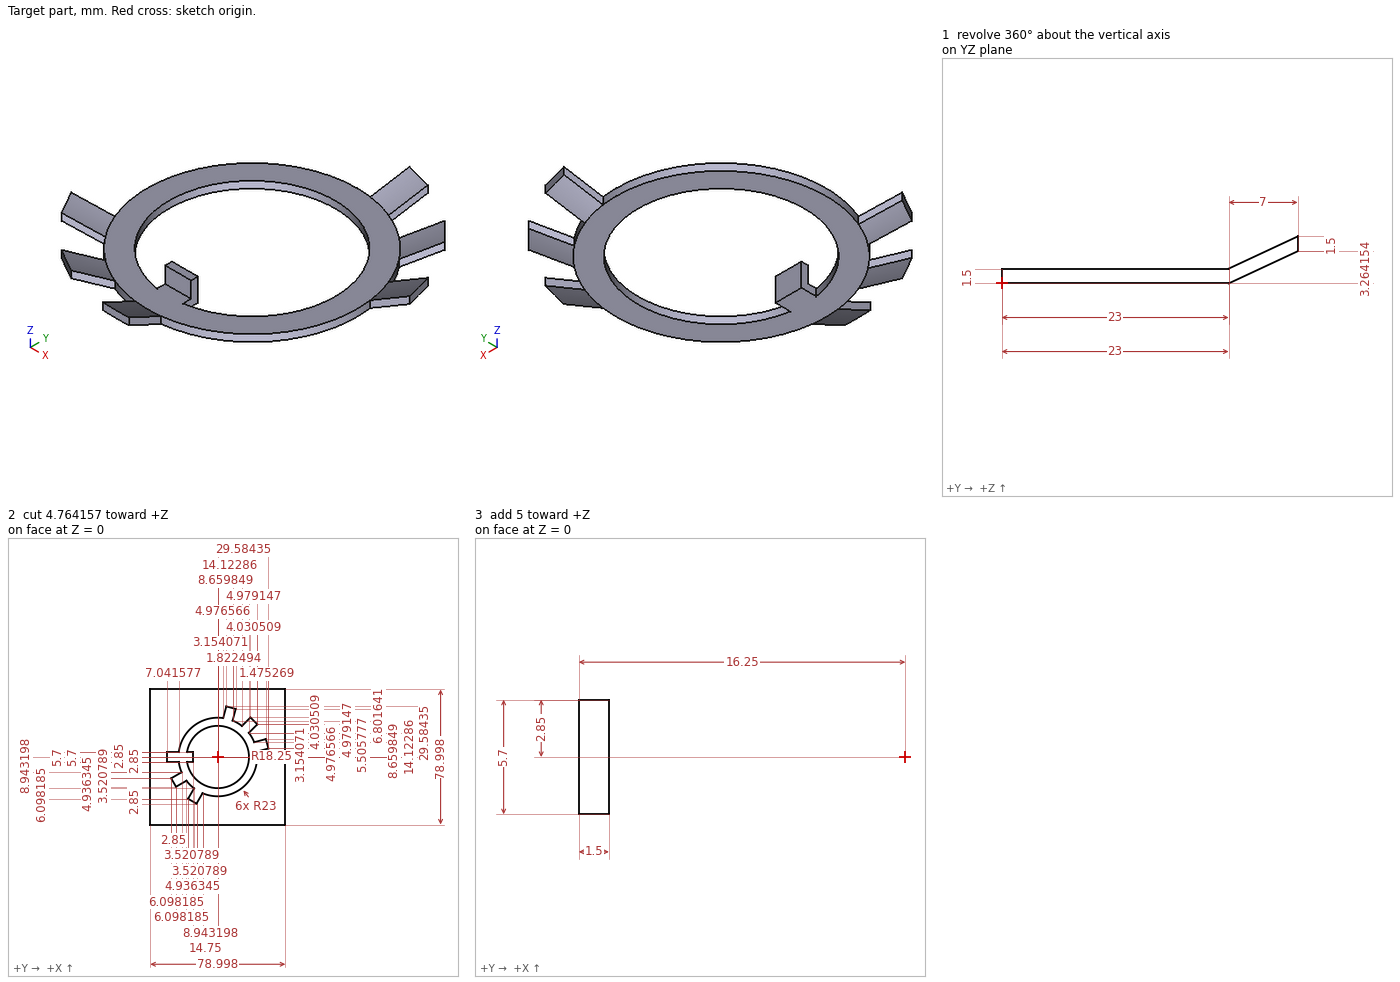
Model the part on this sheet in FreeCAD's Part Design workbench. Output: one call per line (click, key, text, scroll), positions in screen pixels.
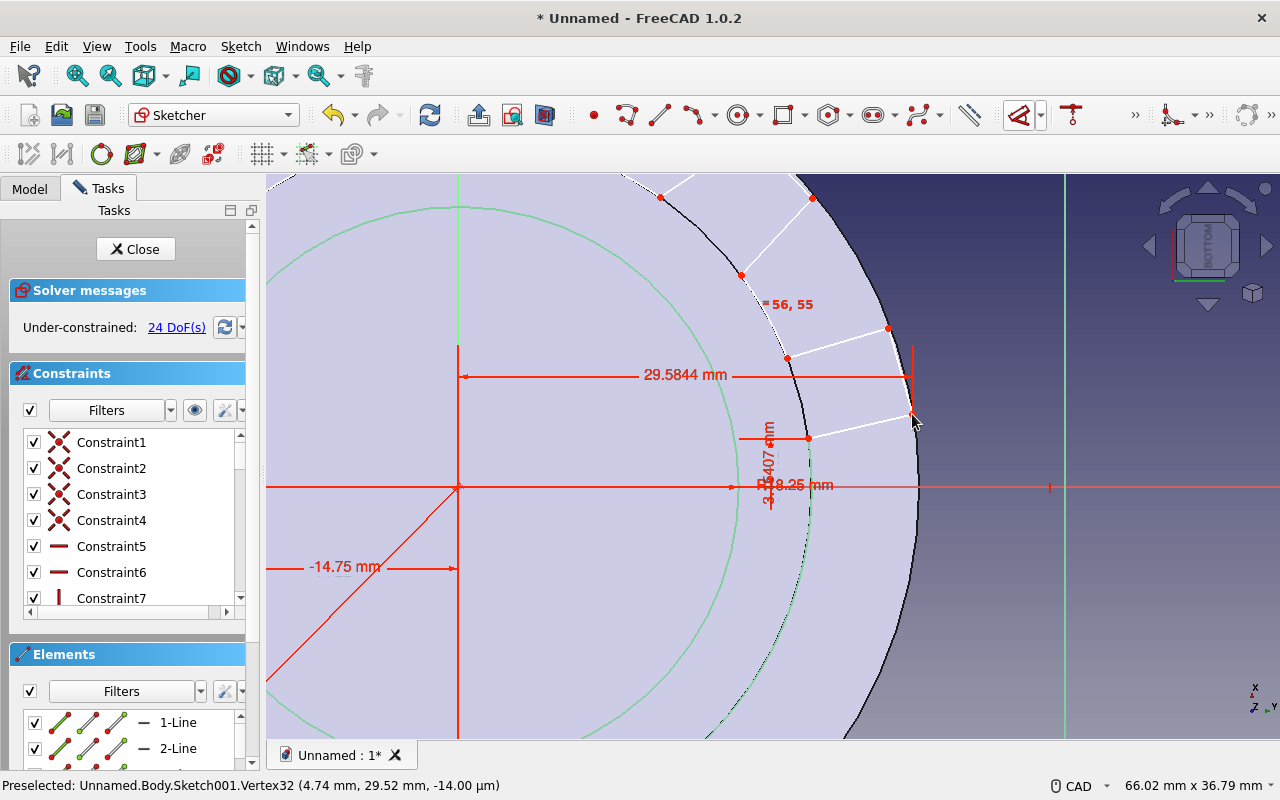
click(913, 414)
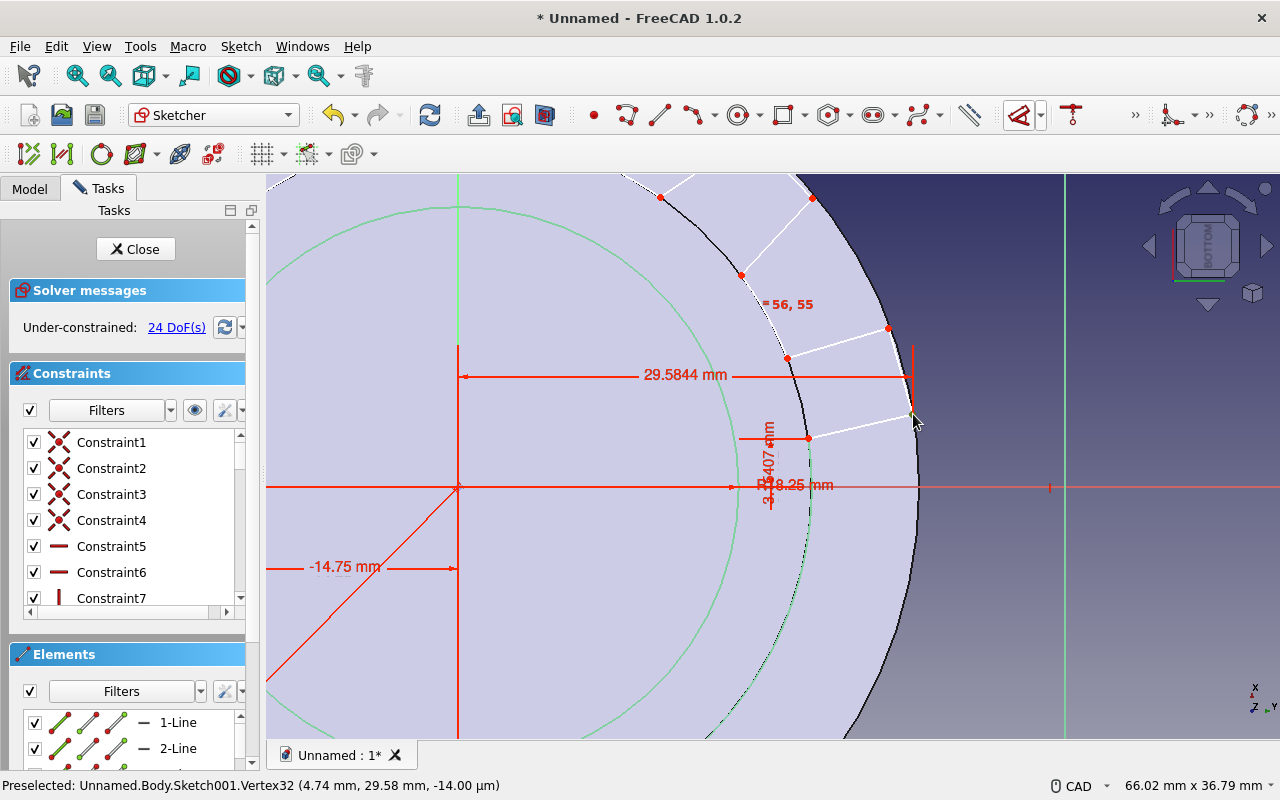
click(1040, 116)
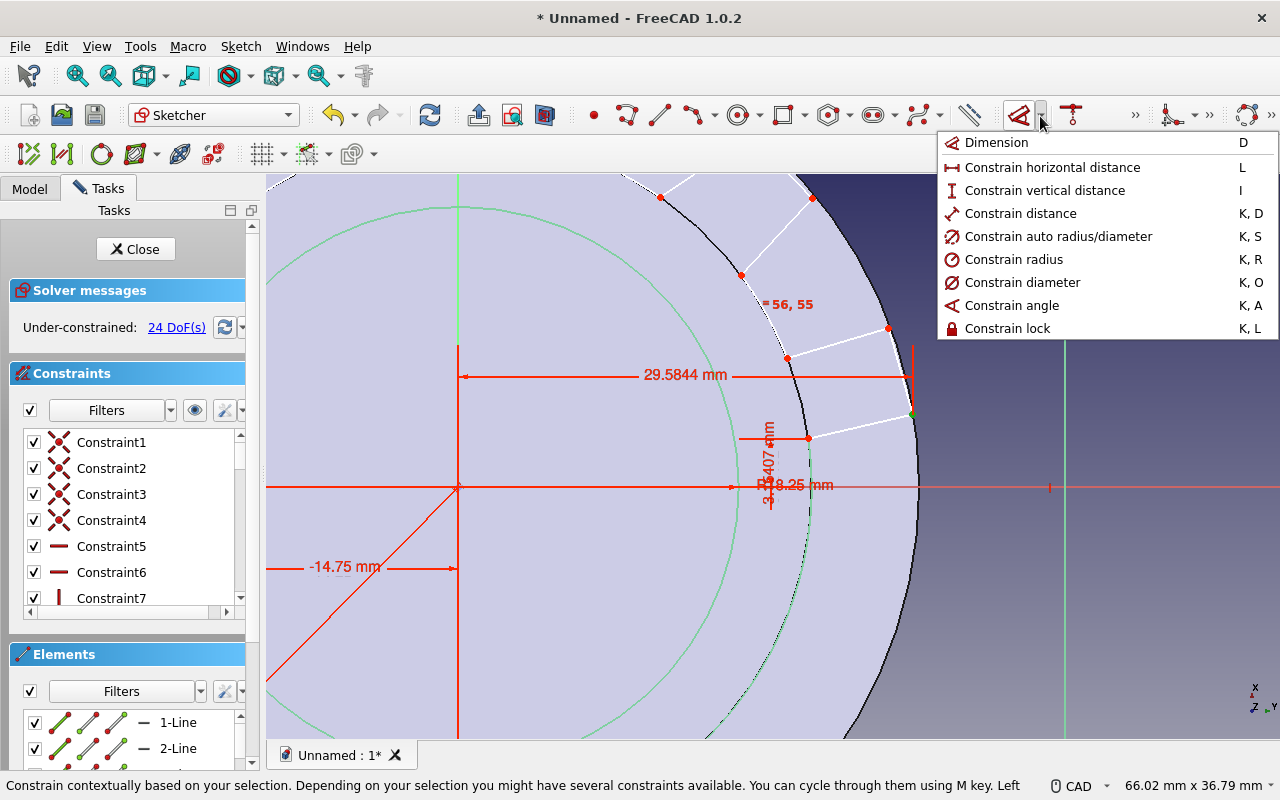
click(1108, 190)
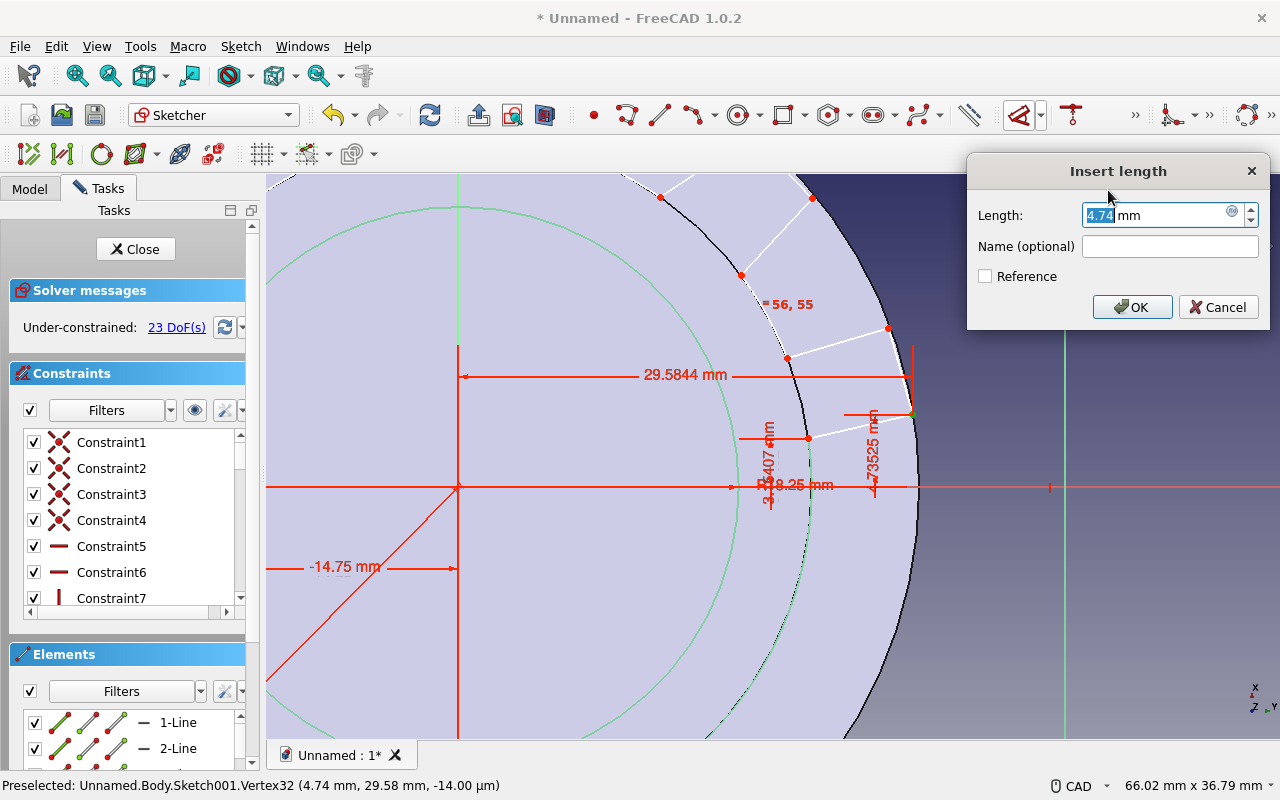
text(4.976566)
key(Return)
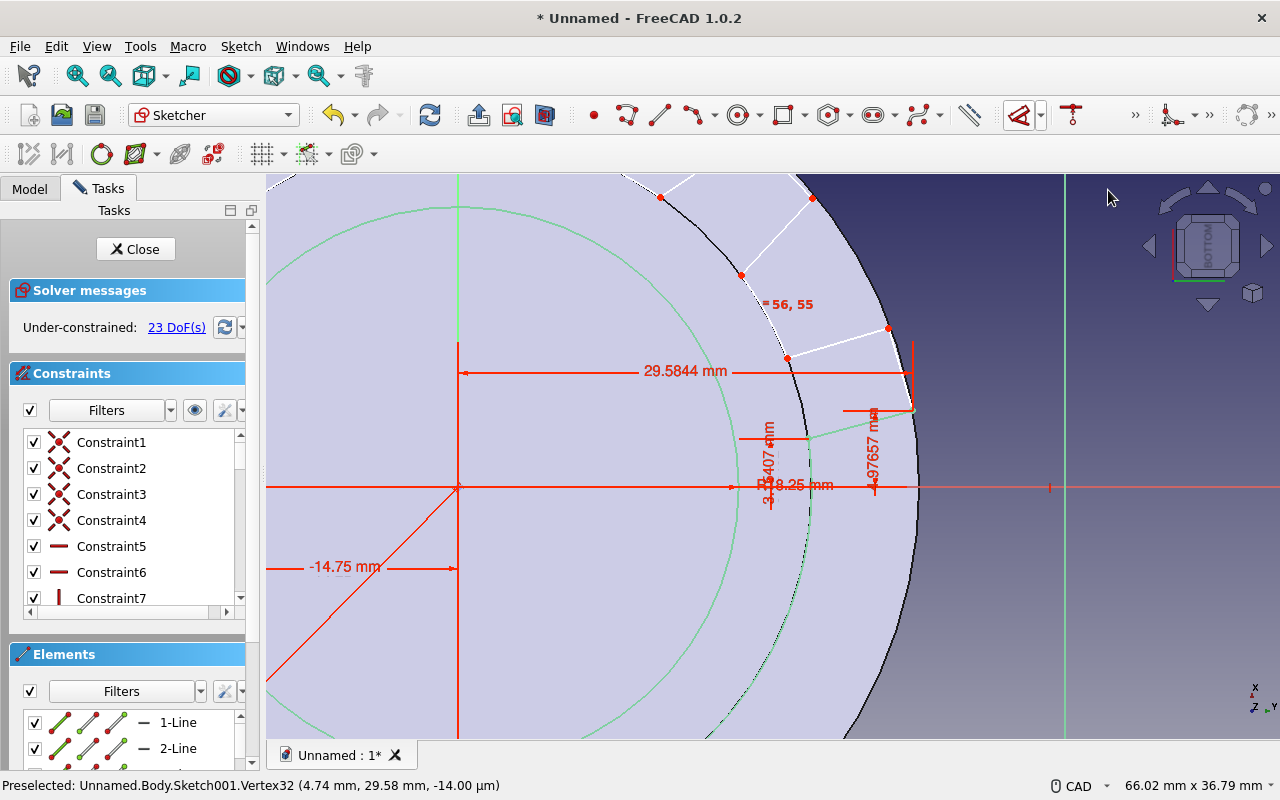
click(787, 358)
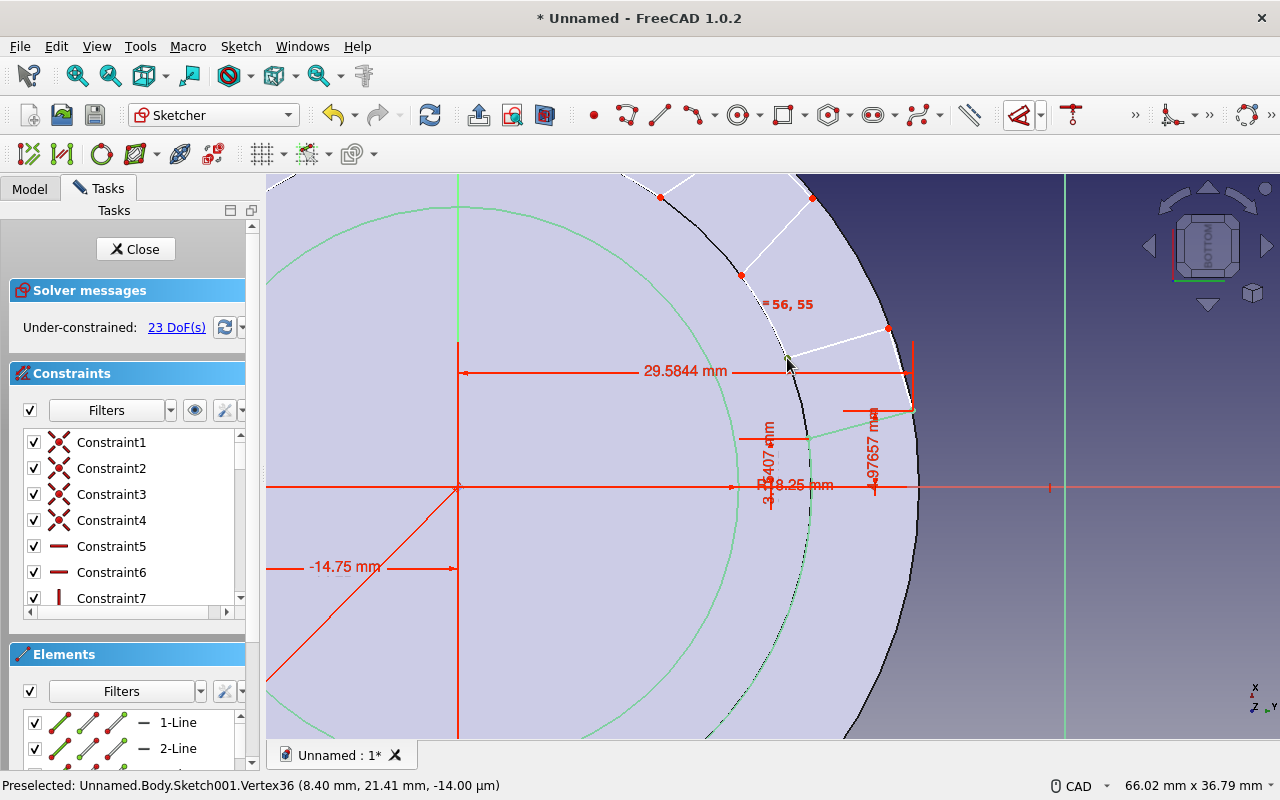
click(1040, 116)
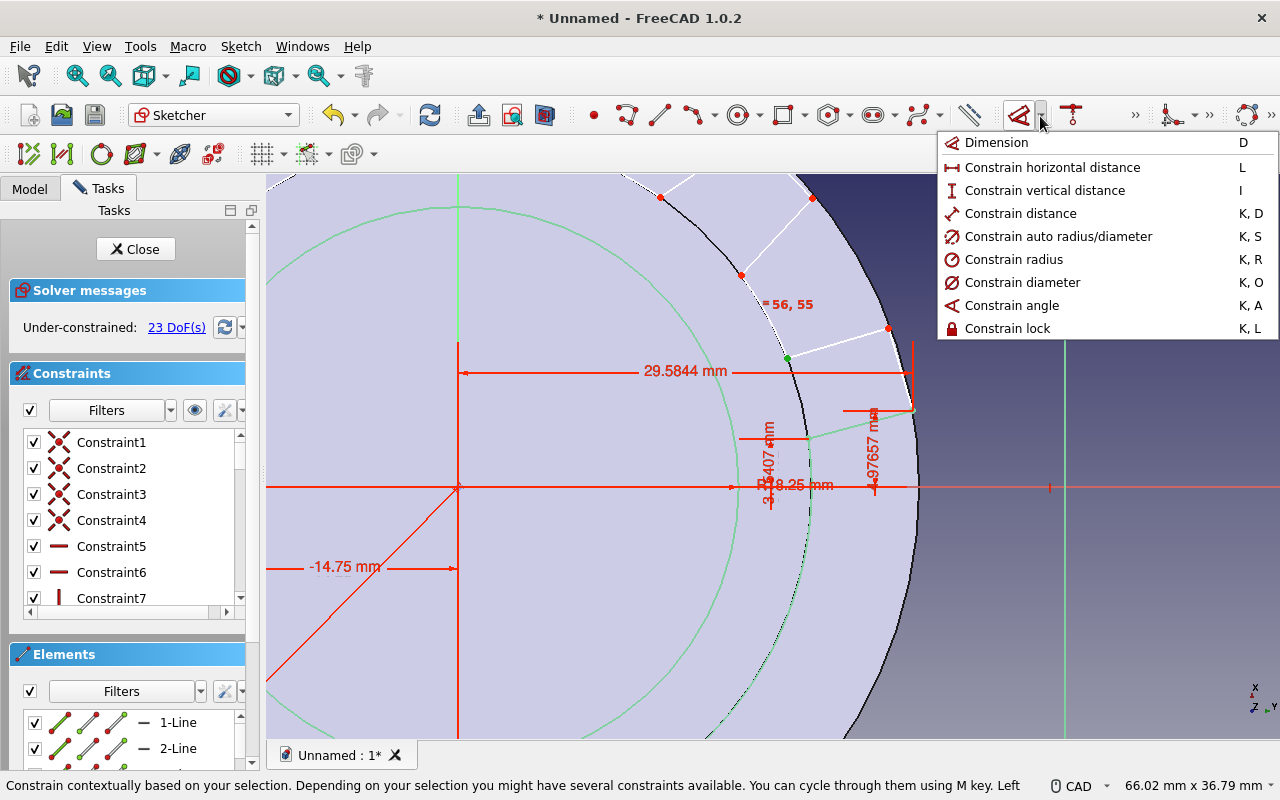
click(1108, 190)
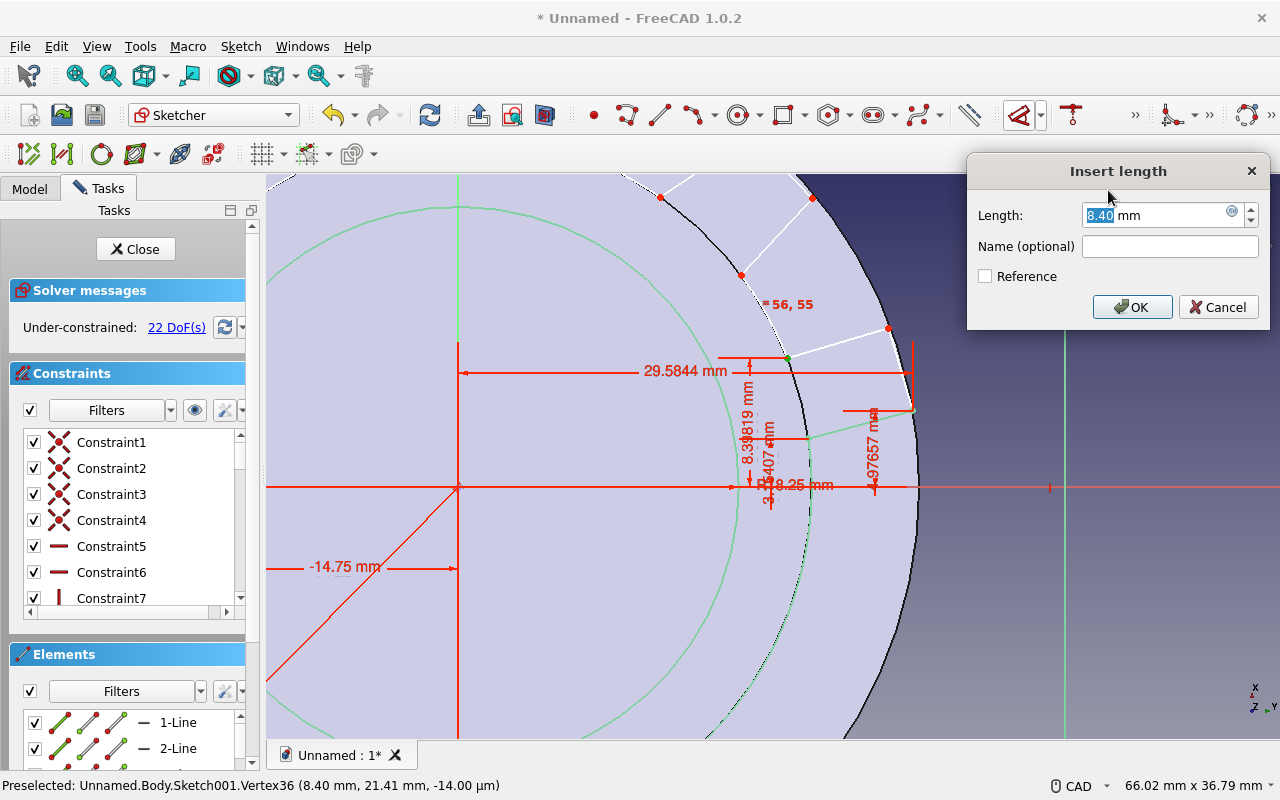
text(8.659849)
key(Return)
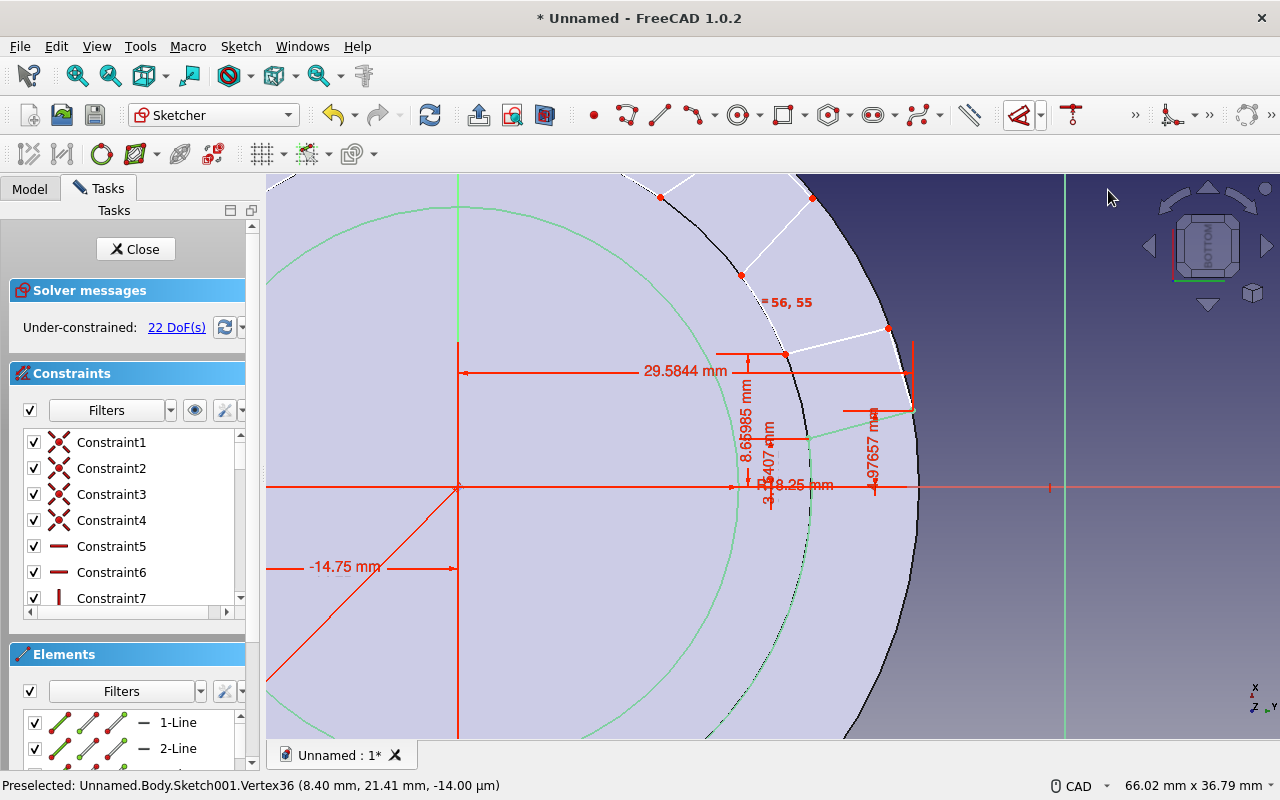
click(741, 275)